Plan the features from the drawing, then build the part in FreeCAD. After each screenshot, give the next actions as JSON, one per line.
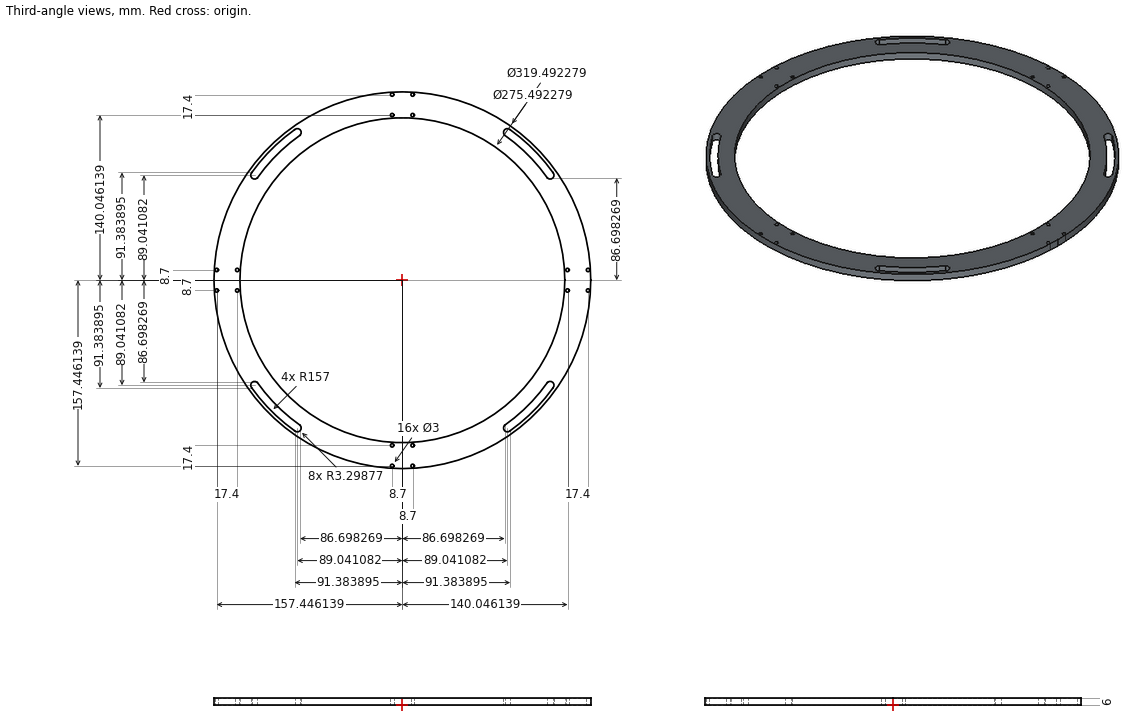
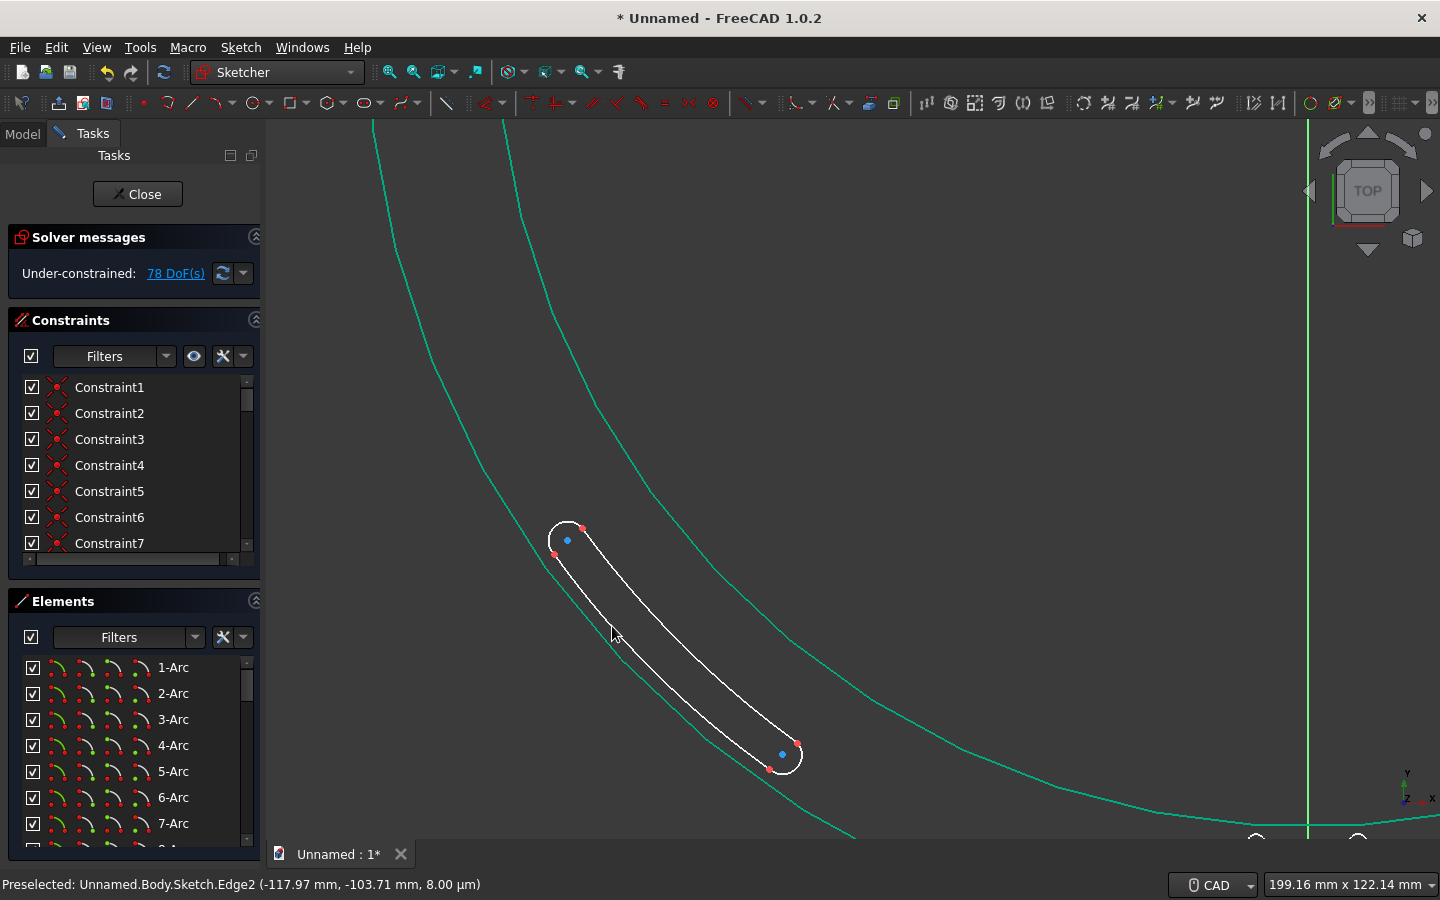
{"action": "left_click", "coordinate": [644, 683]}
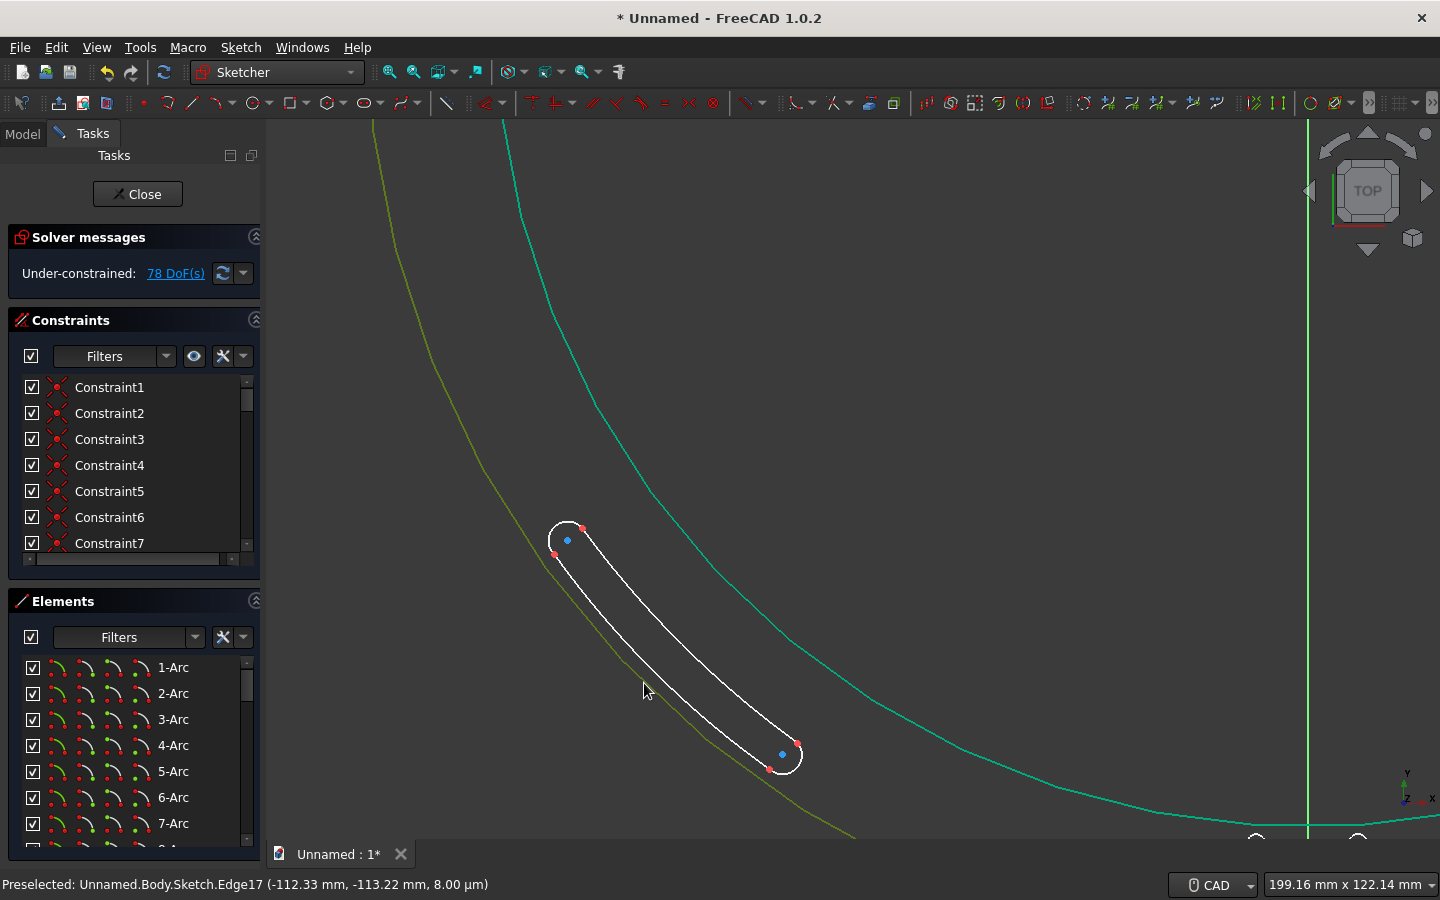
{"action": "left_click", "coordinate": [640, 600]}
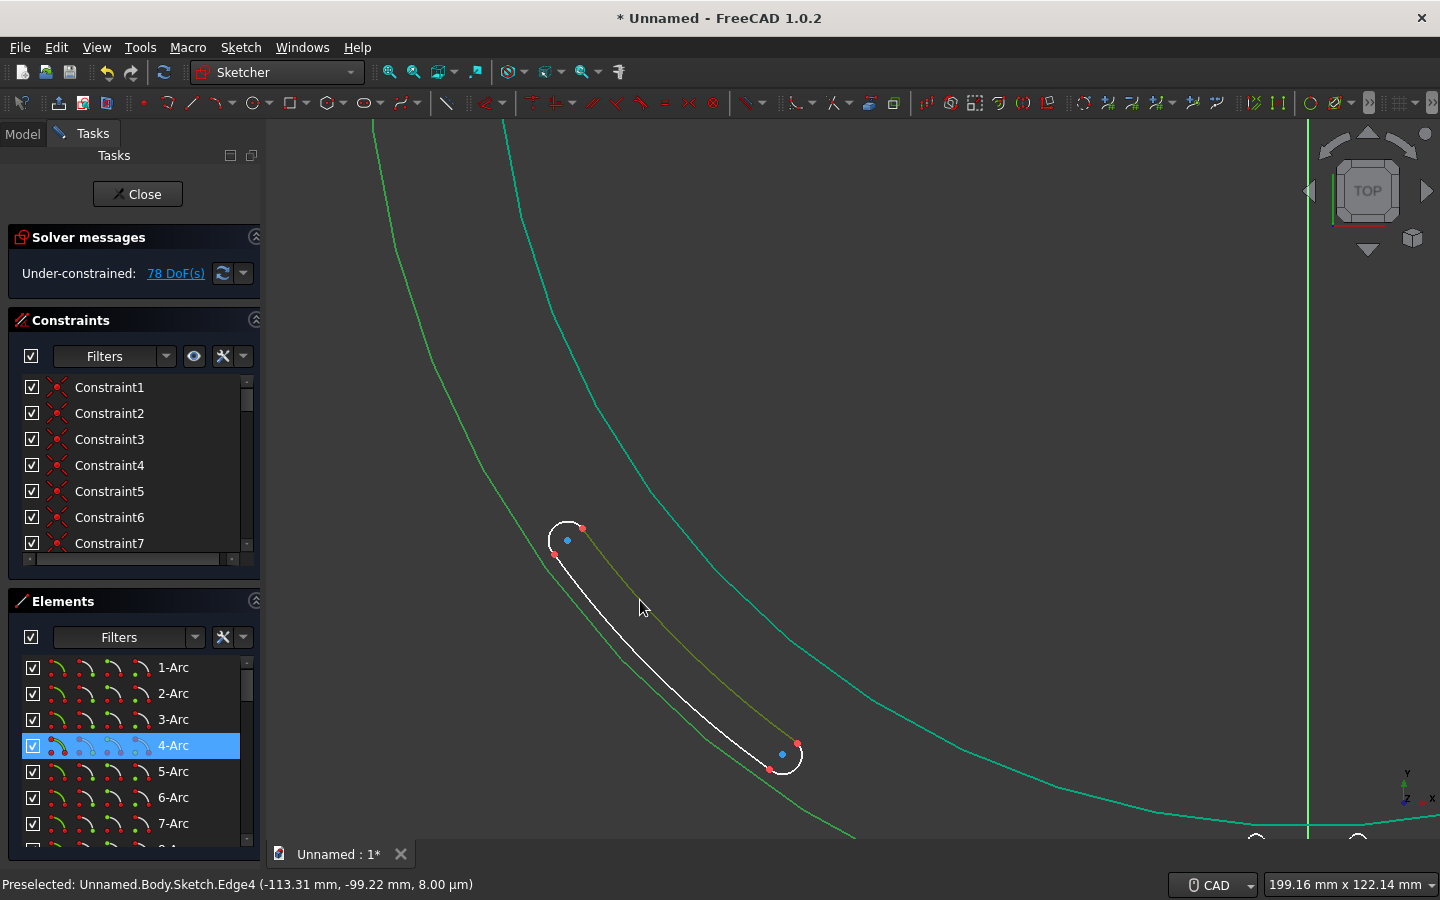
{"action": "key", "text": "c"}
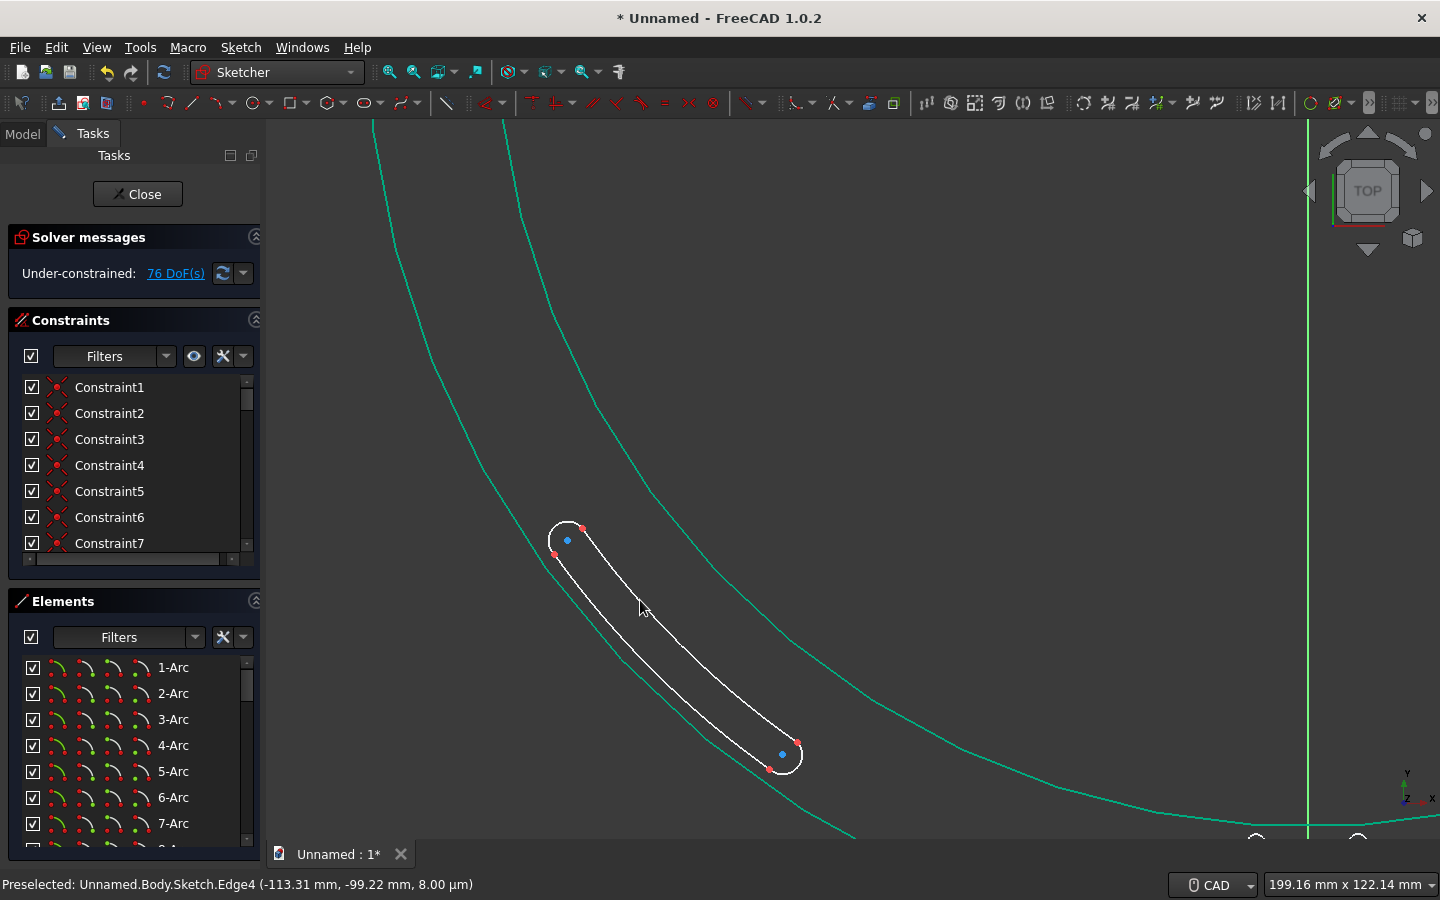
{"action": "left_click", "coordinate": [644, 683]}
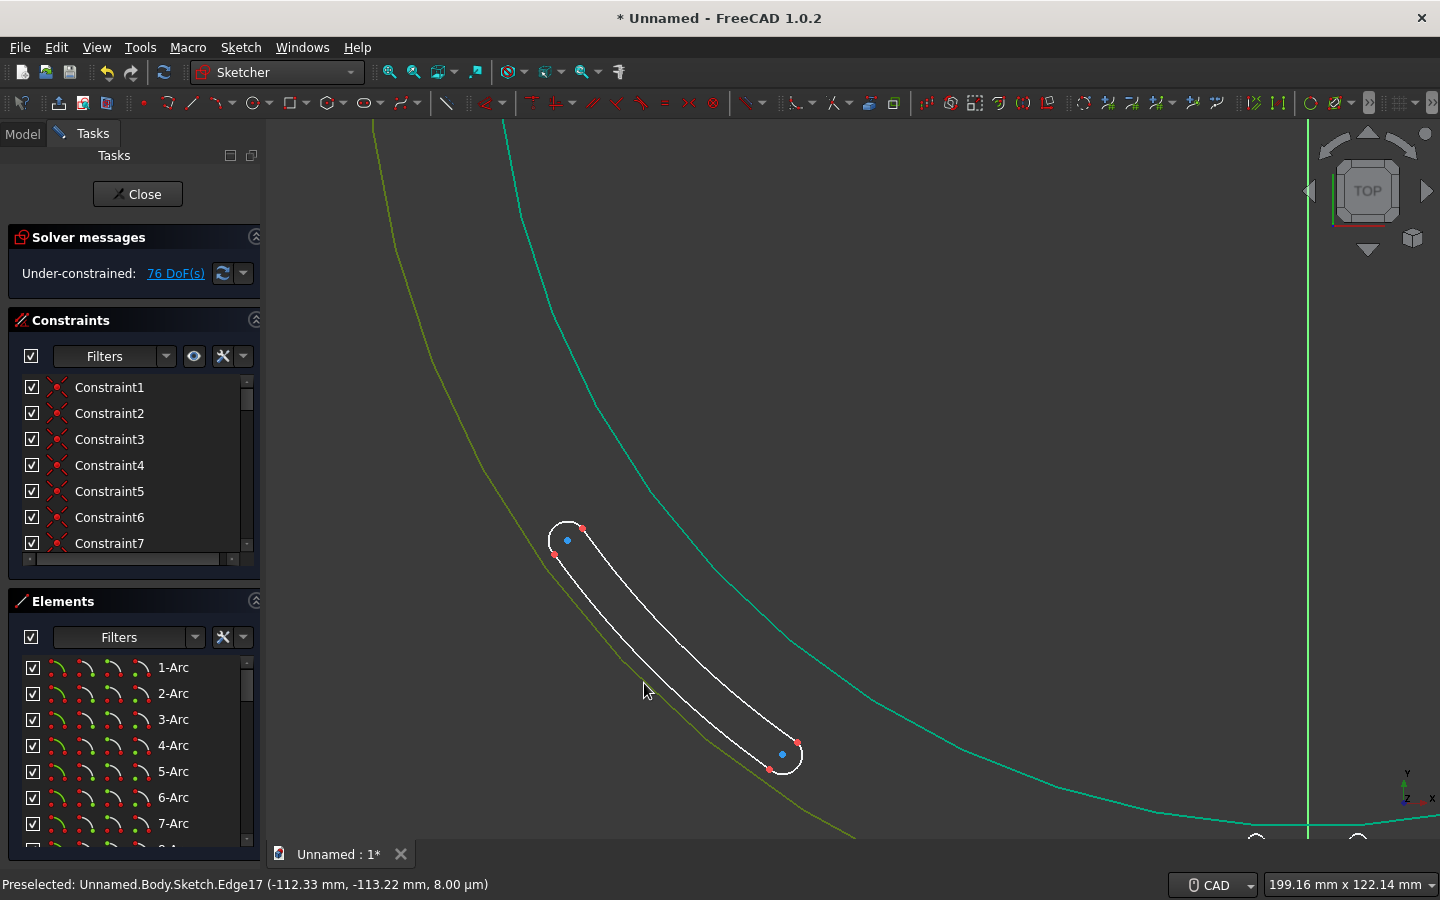
{"action": "scroll", "coordinate": [613, 631], "scroll_direction": "down", "scroll_amount": 7}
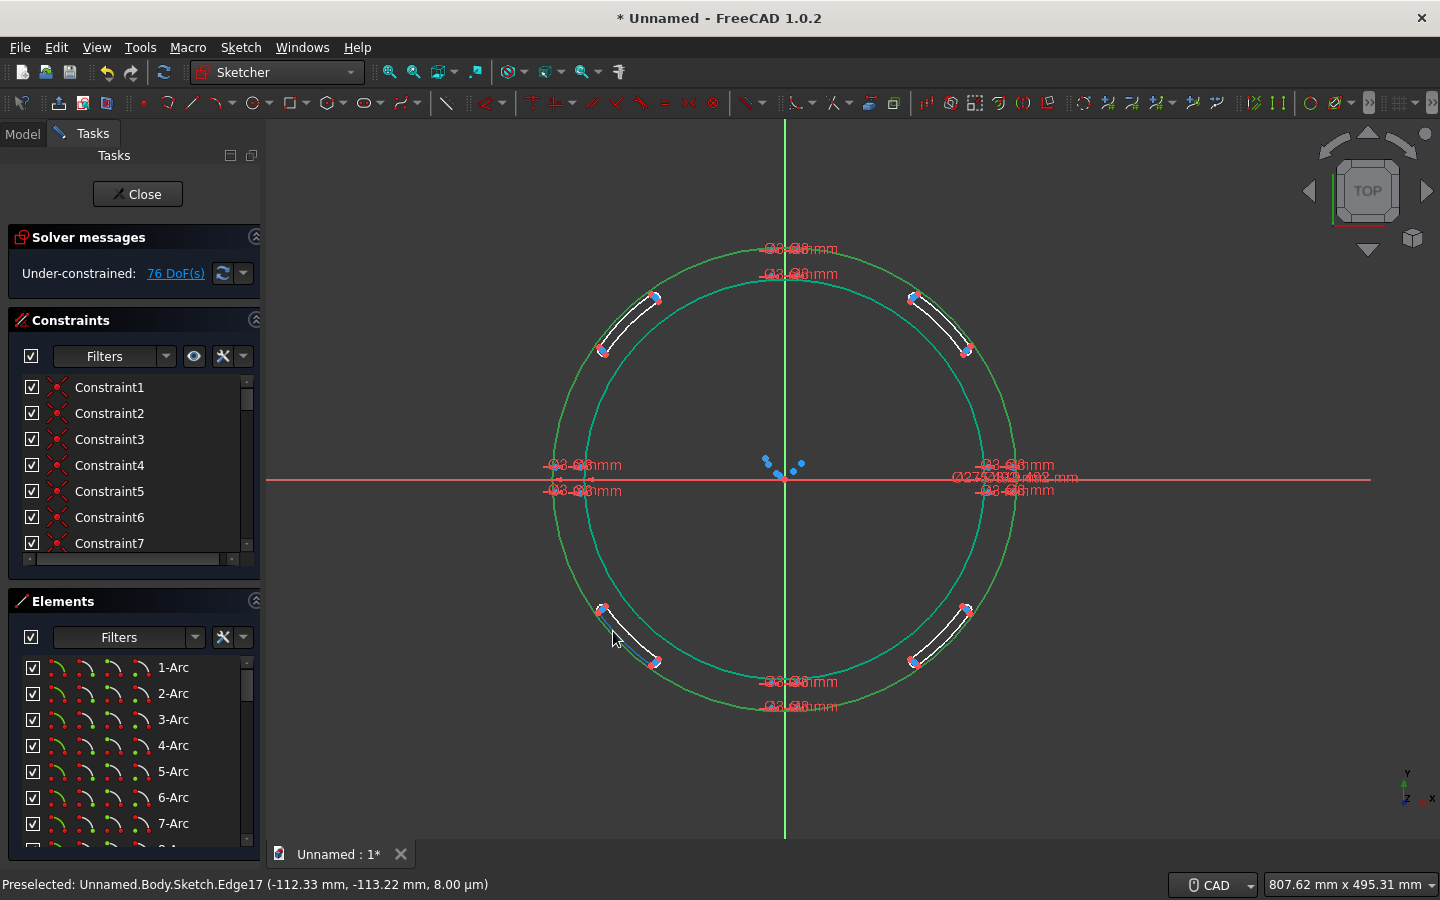
{"action": "scroll", "coordinate": [935, 652], "scroll_direction": "up", "scroll_amount": 7}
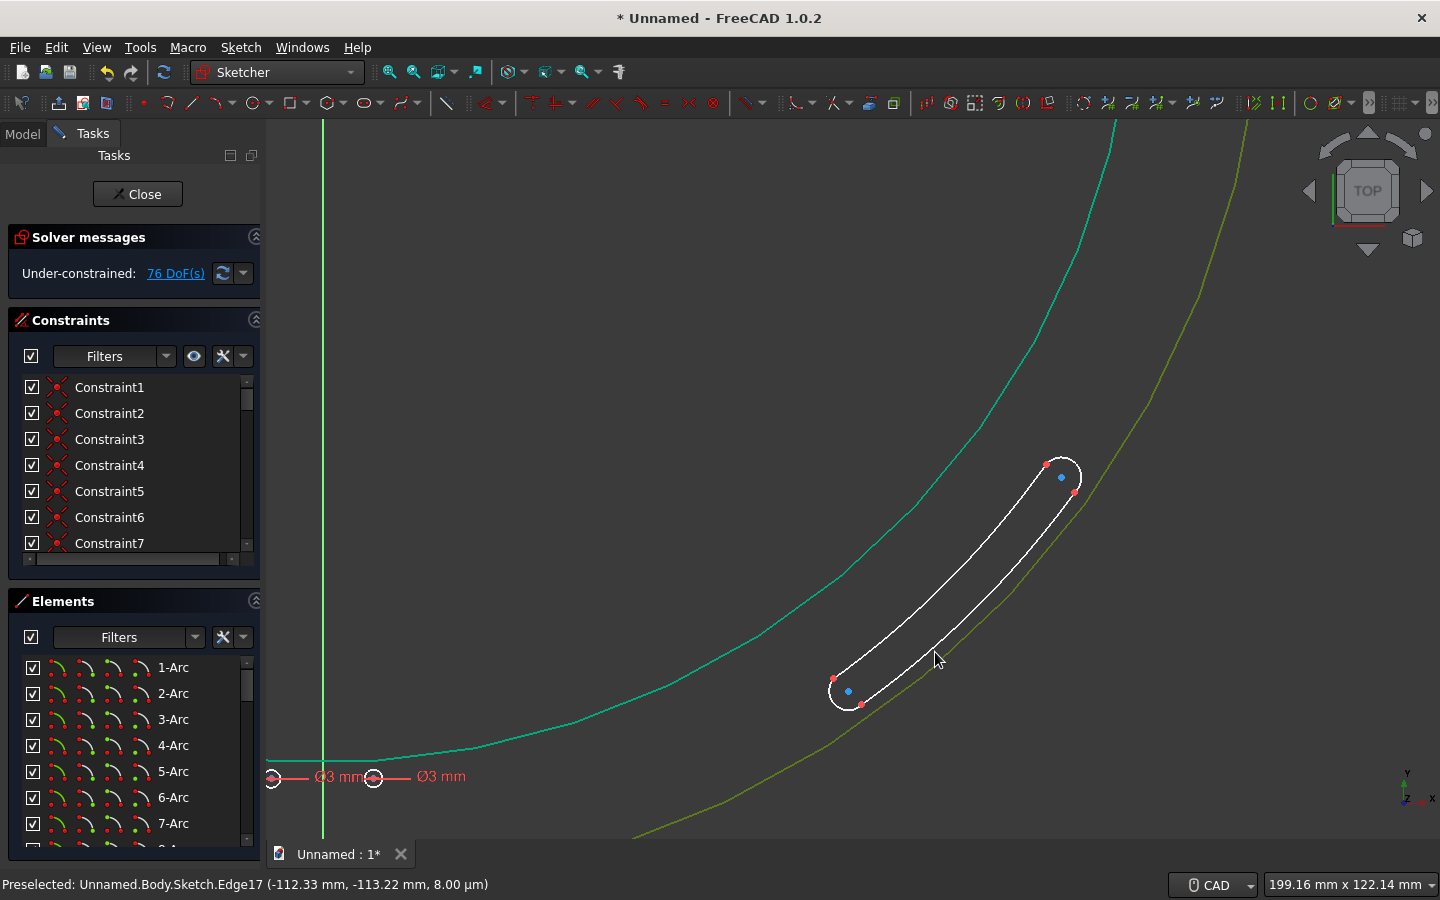
{"action": "left_click", "coordinate": [932, 649]}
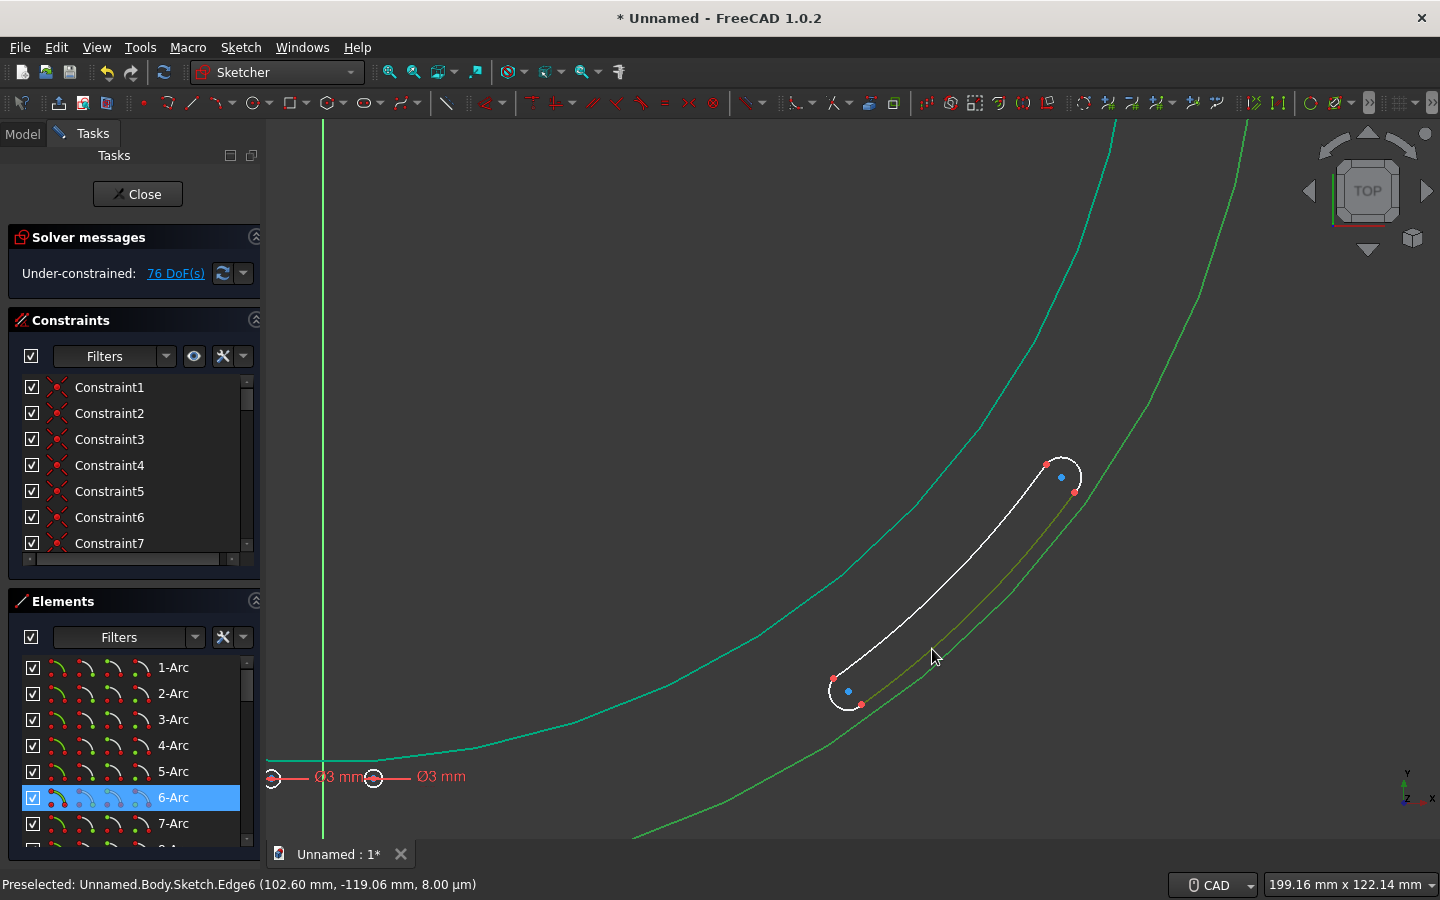
{"action": "key", "text": "c"}